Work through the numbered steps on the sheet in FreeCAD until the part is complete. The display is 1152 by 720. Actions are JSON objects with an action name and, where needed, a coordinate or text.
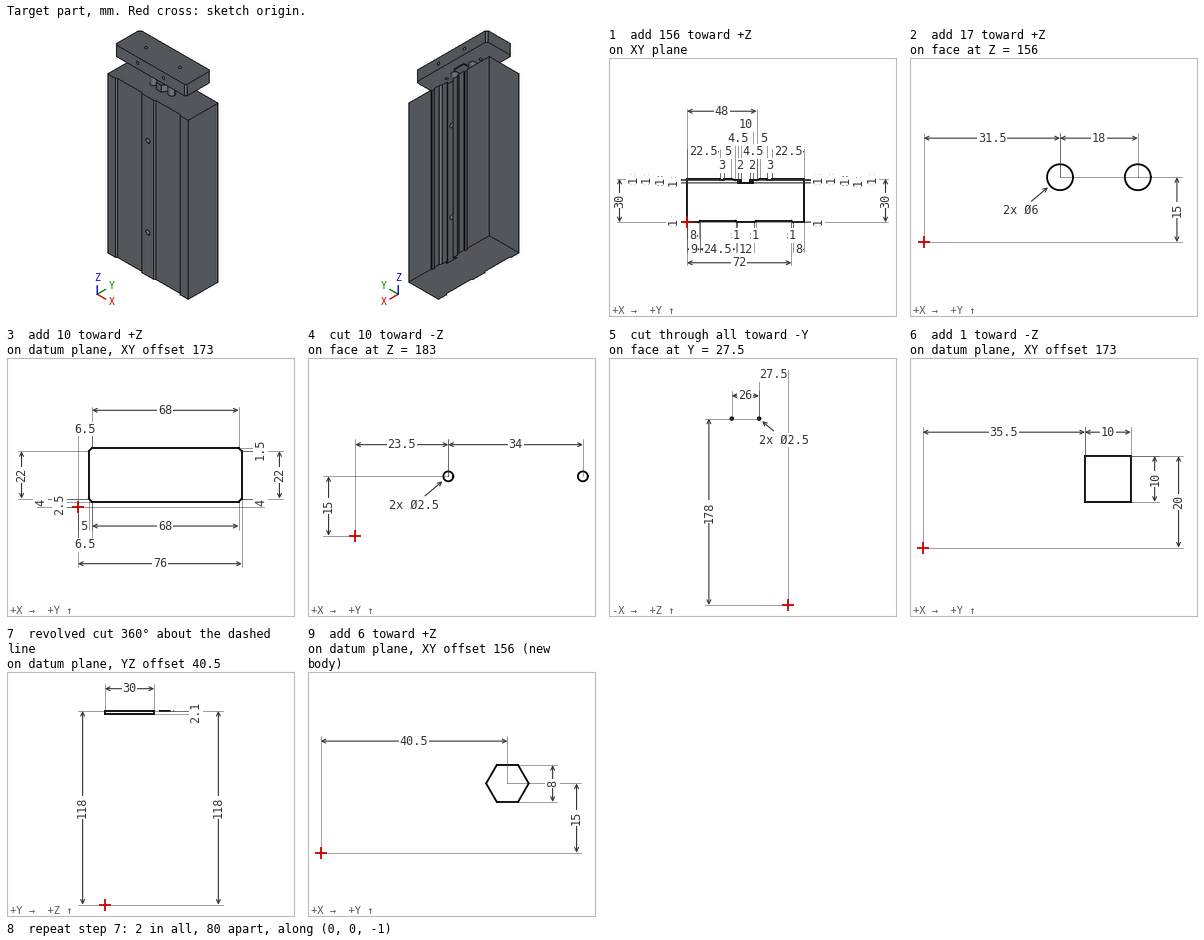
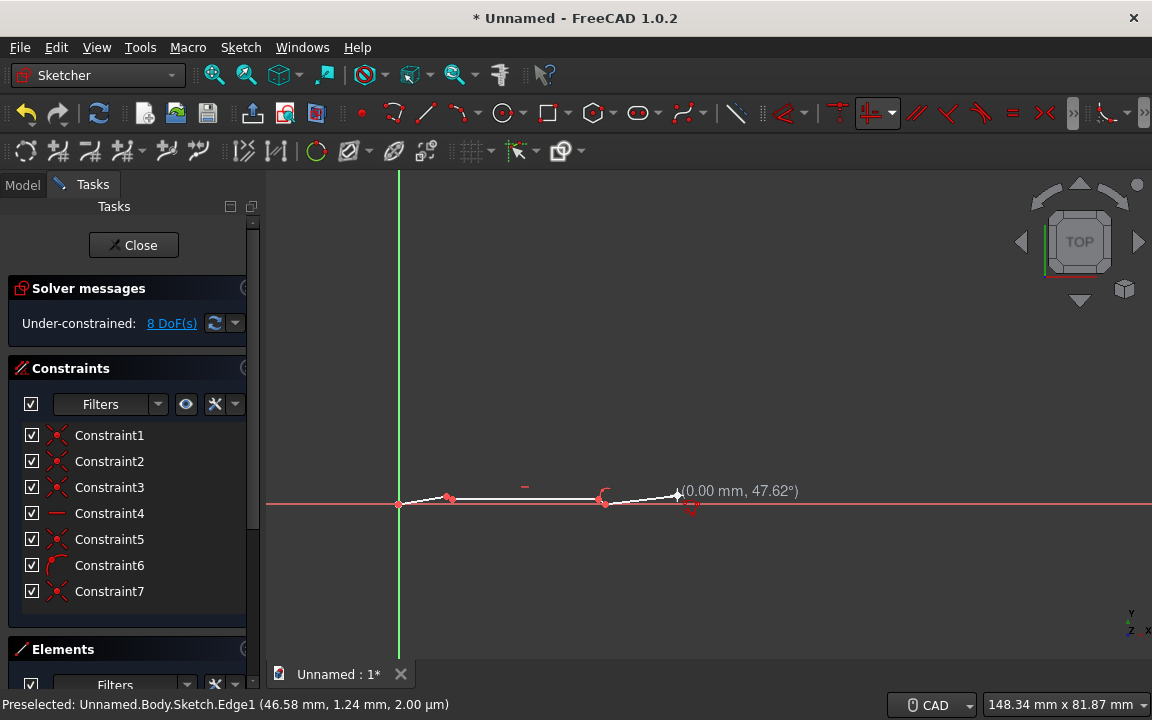
{"action": "scroll", "coordinate": [683, 499], "scroll_direction": "up", "scroll_amount": 5}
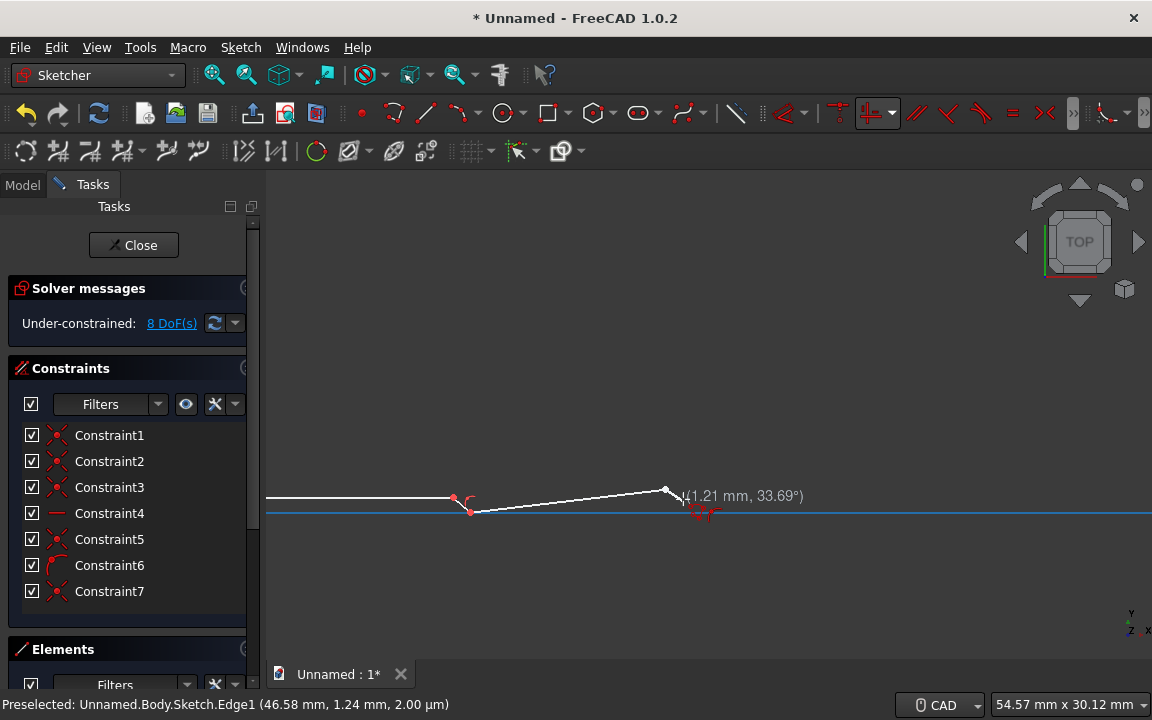
{"action": "left_click", "coordinate": [681, 497]}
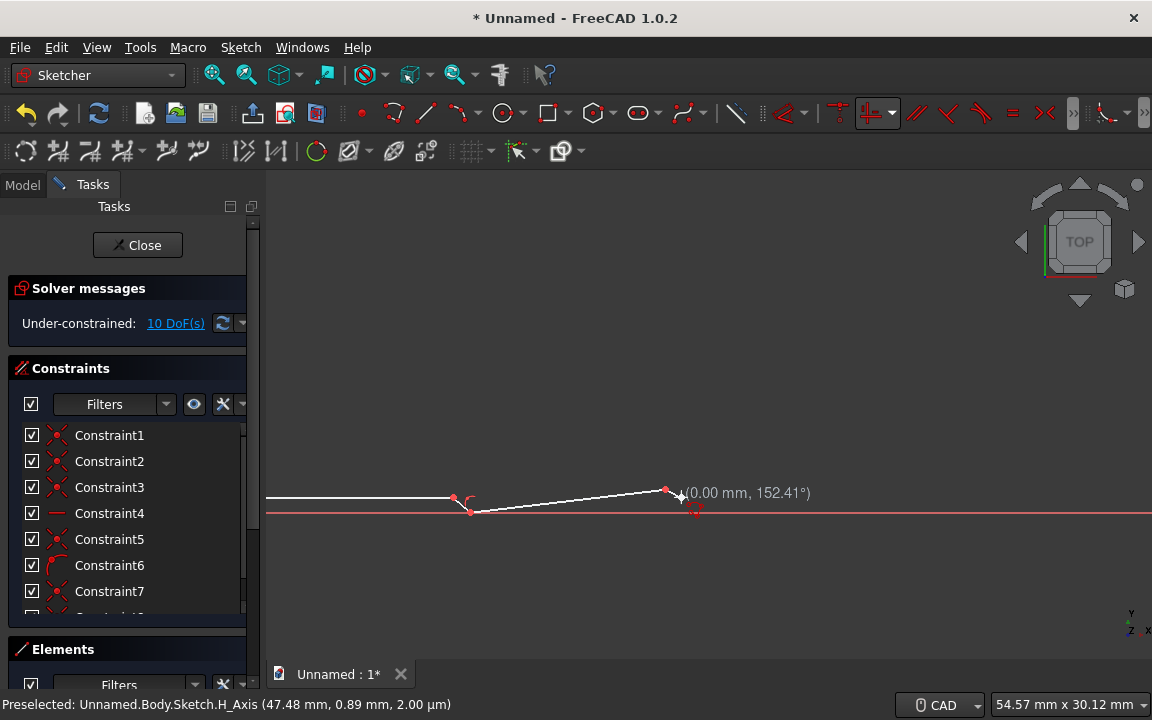
{"action": "scroll", "coordinate": [683, 499], "scroll_direction": "down", "scroll_amount": 5}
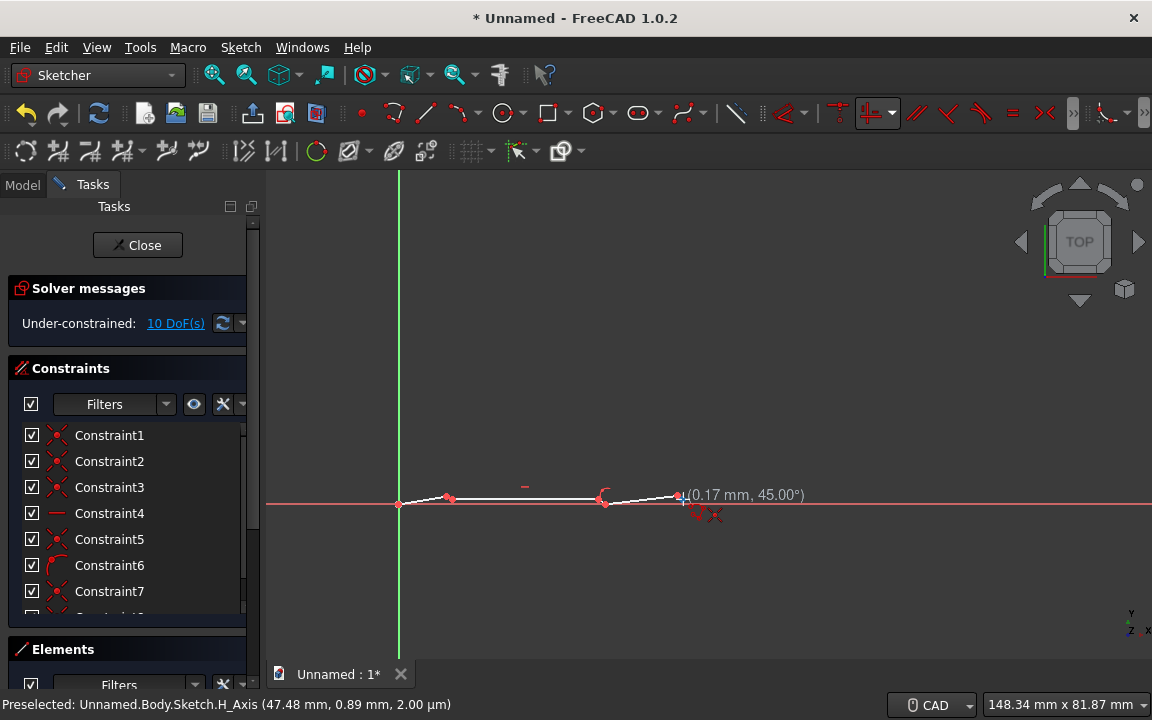
{"action": "scroll", "coordinate": [829, 499], "scroll_direction": "up", "scroll_amount": 5}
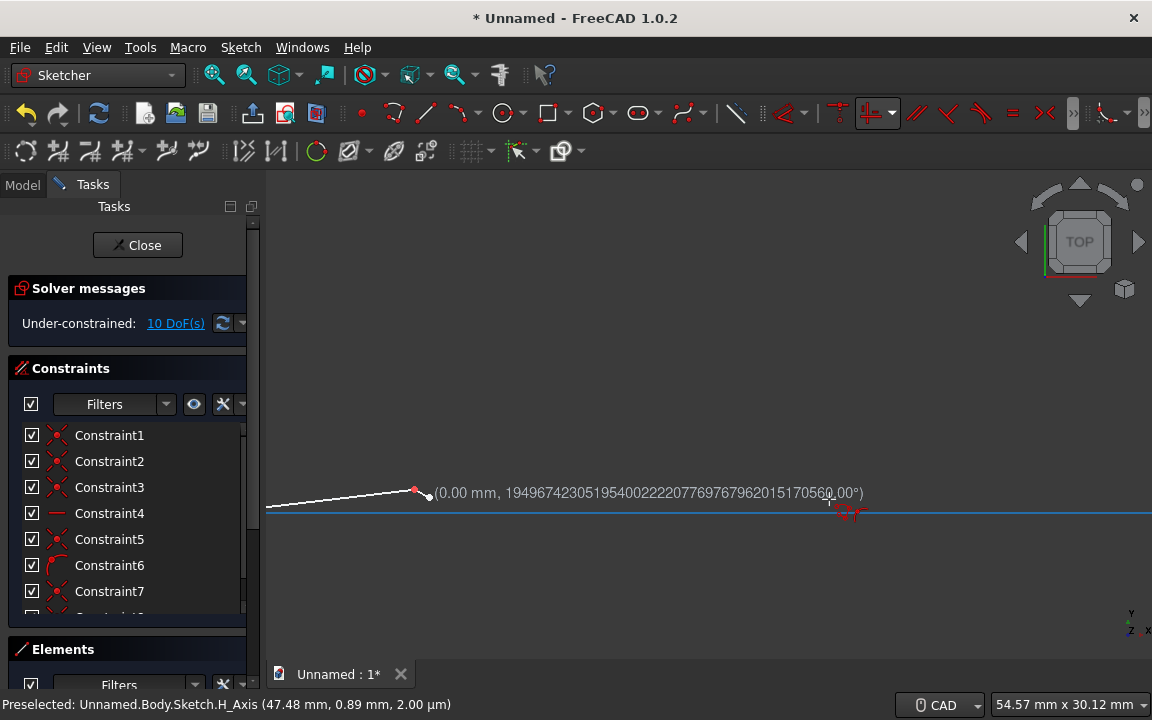
{"action": "left_click", "coordinate": [828, 497]}
{"action": "left_click", "coordinate": [844, 513]}
{"action": "left_click", "coordinate": [974, 504]}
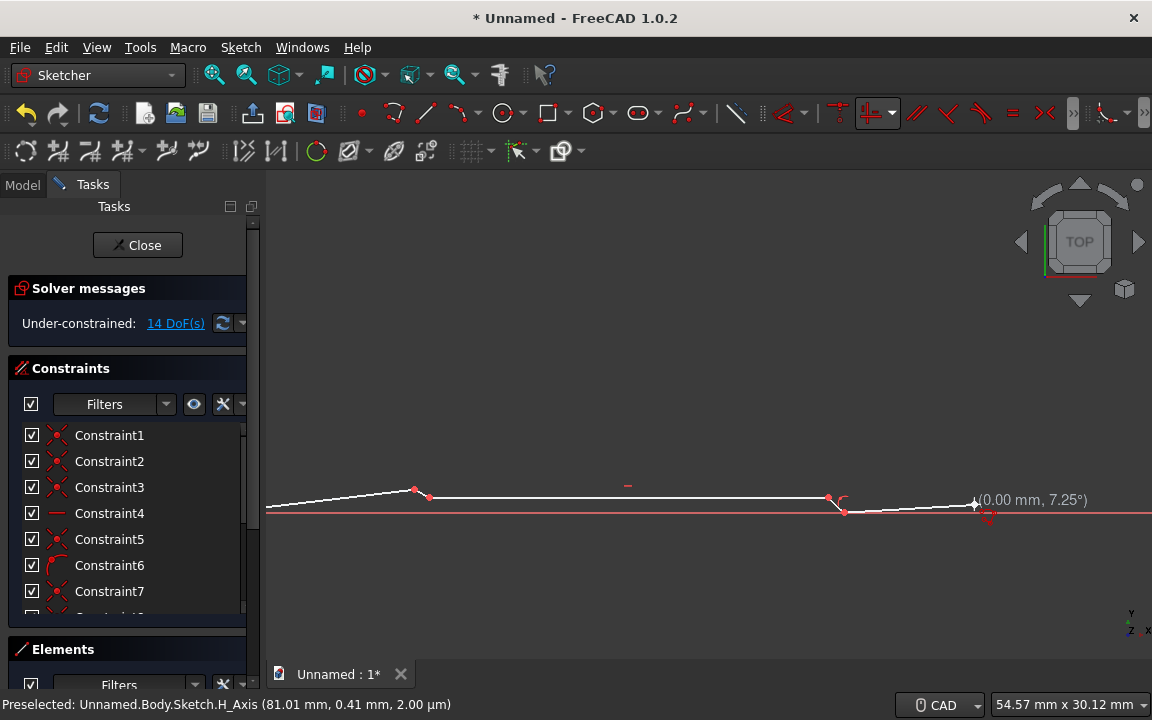
{"action": "scroll", "coordinate": [829, 499], "scroll_direction": "down", "scroll_amount": 5}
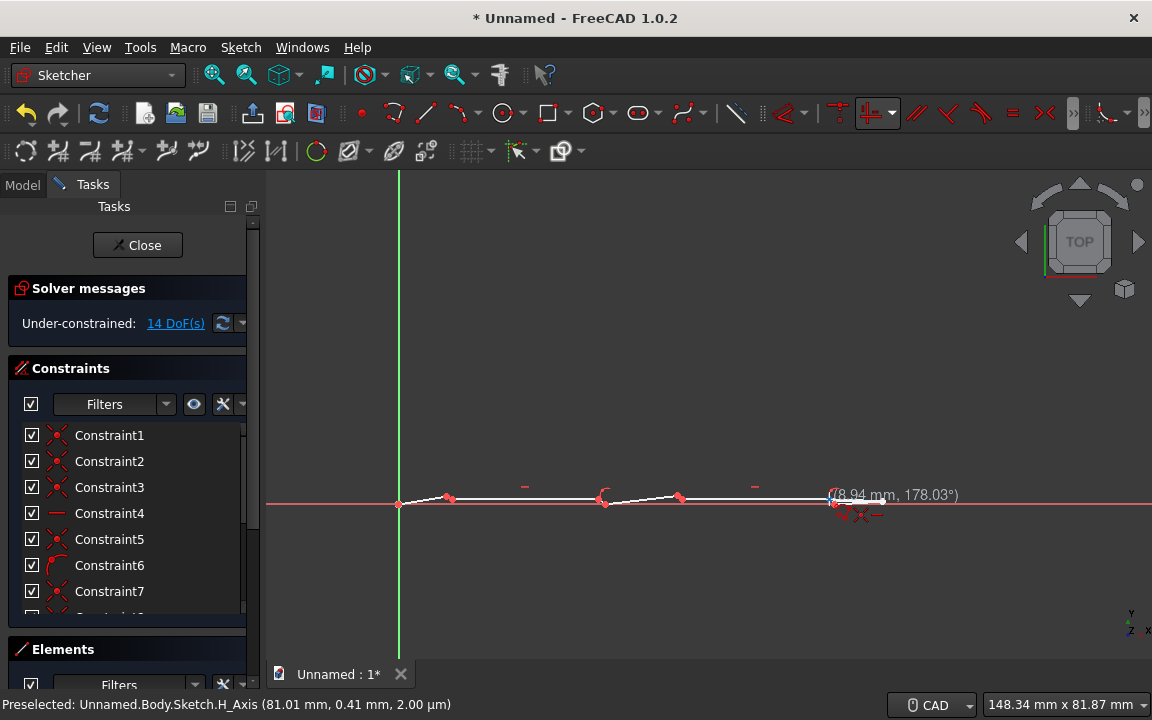
{"action": "left_click", "coordinate": [883, 325]}
{"action": "left_click", "coordinate": [748, 325]}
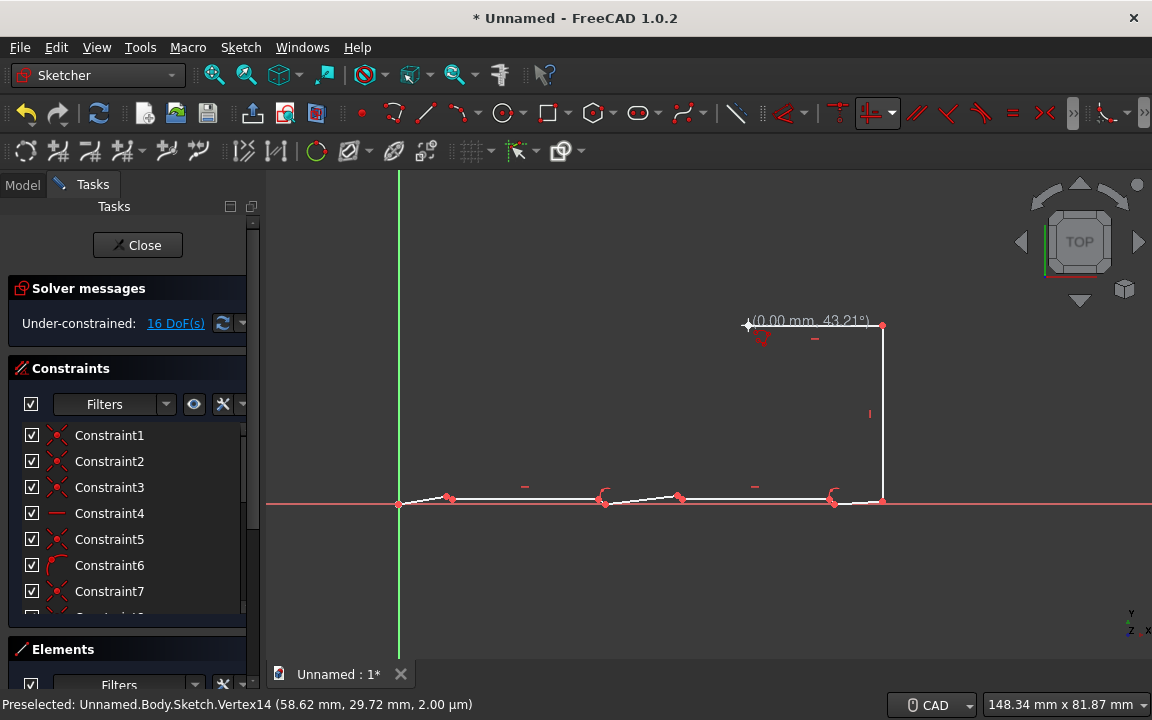
{"action": "scroll", "coordinate": [748, 331], "scroll_direction": "up", "scroll_amount": 5}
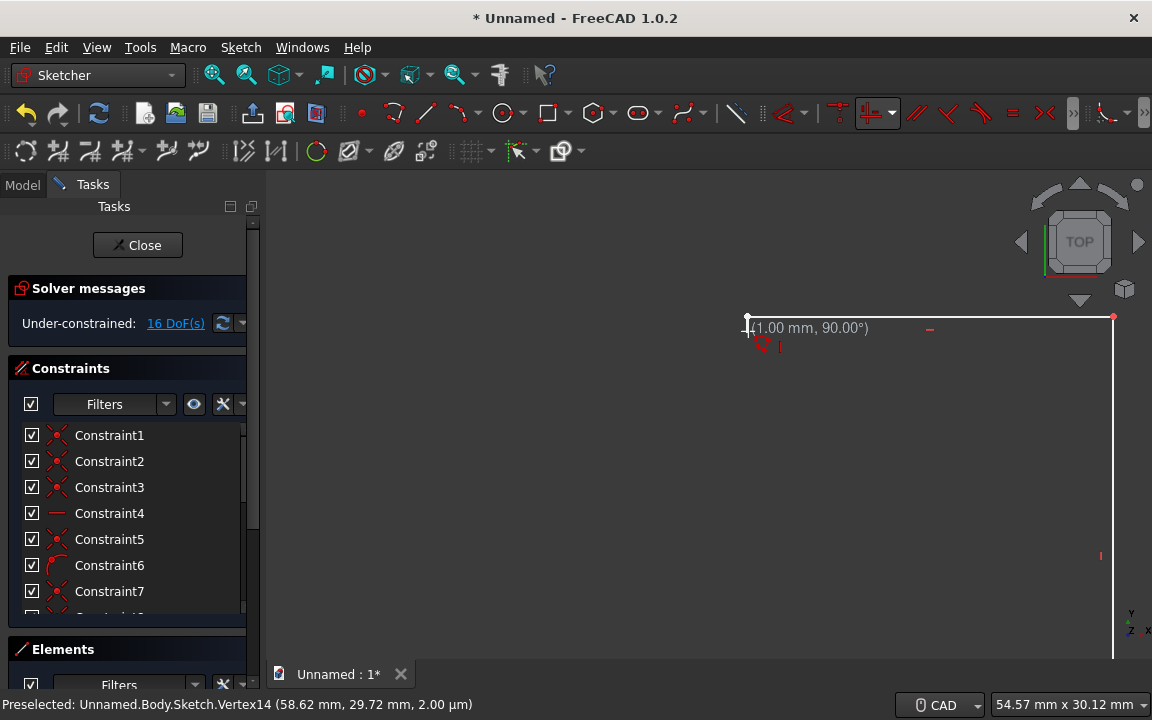
{"action": "left_click", "coordinate": [747, 331]}
{"action": "left_click", "coordinate": [699, 331]}
{"action": "left_click", "coordinate": [699, 315]}
{"action": "left_click", "coordinate": [618, 315]}
{"action": "left_click", "coordinate": [577, 331]}
{"action": "left_click", "coordinate": [504, 331]}
{"action": "left_click", "coordinate": [504, 347]}
{"action": "left_click", "coordinate": [537, 347]}
{"action": "left_click", "coordinate": [537, 364]}
{"action": "left_click", "coordinate": [374, 364]}
{"action": "left_click", "coordinate": [374, 347]}
{"action": "left_click", "coordinate": [407, 347]}
{"action": "left_click", "coordinate": [407, 331]}
{"action": "left_click", "coordinate": [334, 331]}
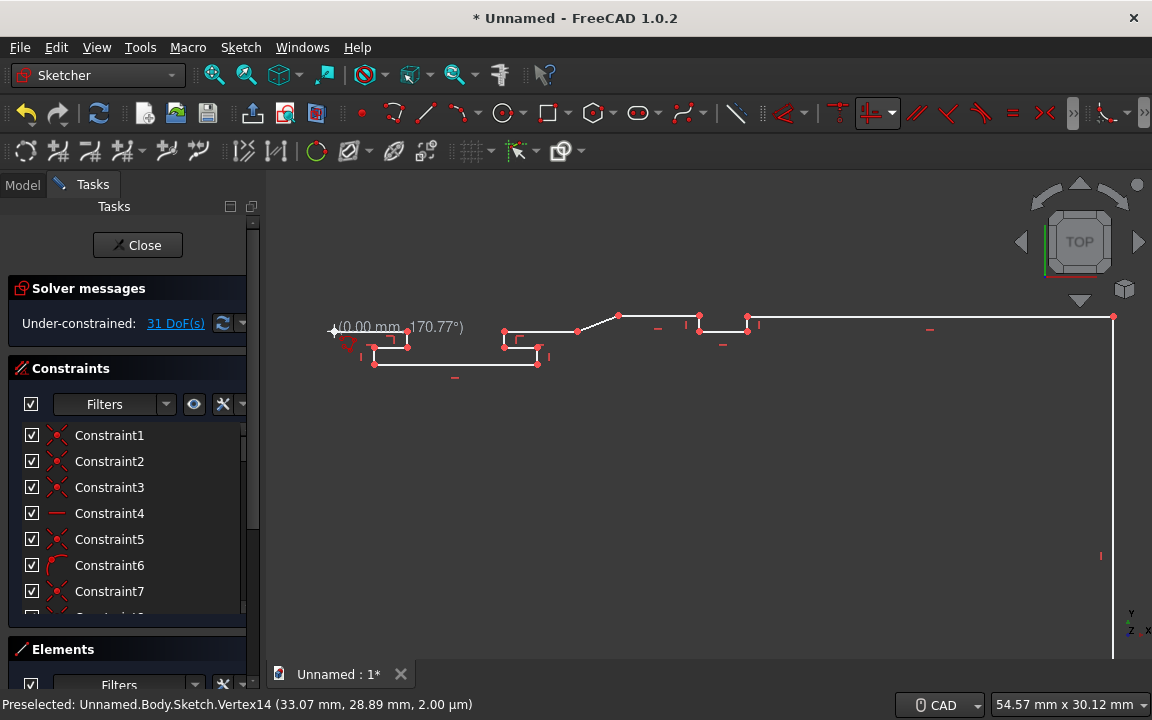
{"action": "scroll", "coordinate": [748, 331], "scroll_direction": "down", "scroll_amount": 5}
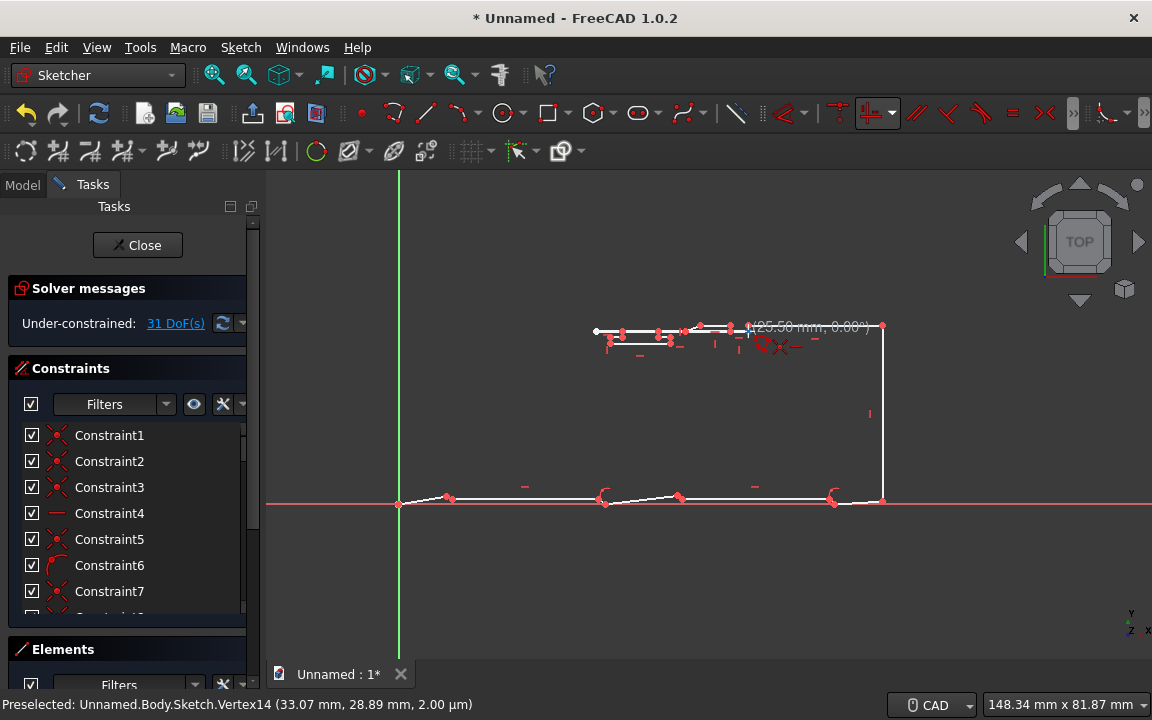
{"action": "left_click", "coordinate": [581, 325]}
{"action": "left_click", "coordinate": [551, 325]}